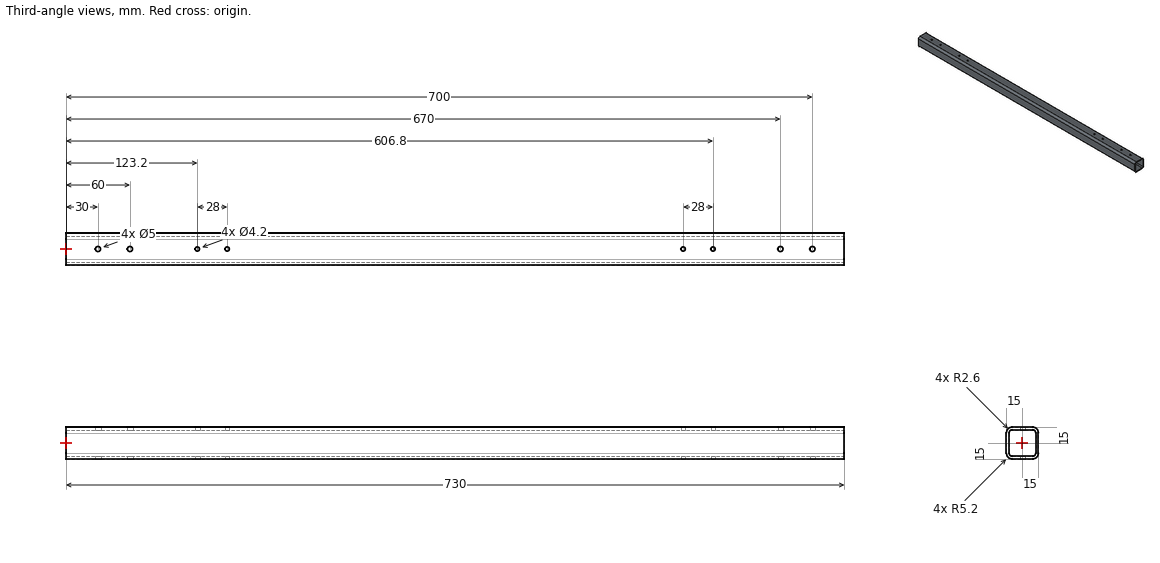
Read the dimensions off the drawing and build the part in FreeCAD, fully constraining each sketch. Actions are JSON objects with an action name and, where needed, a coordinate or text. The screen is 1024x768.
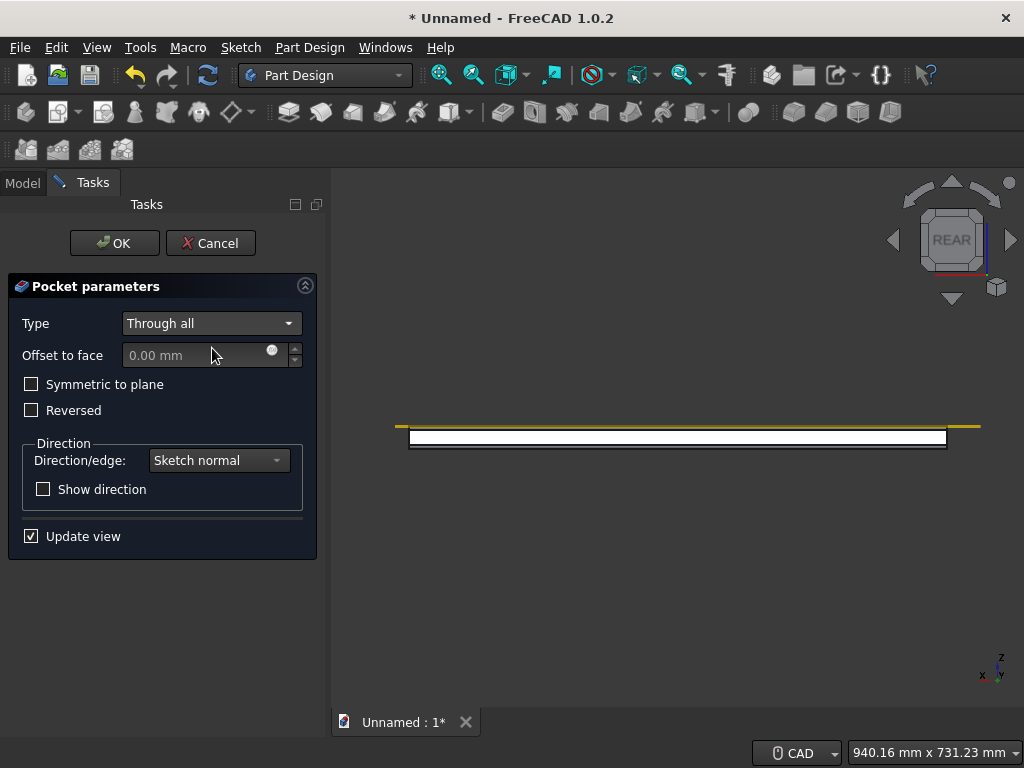
{"action": "left_click", "coordinate": [115, 243]}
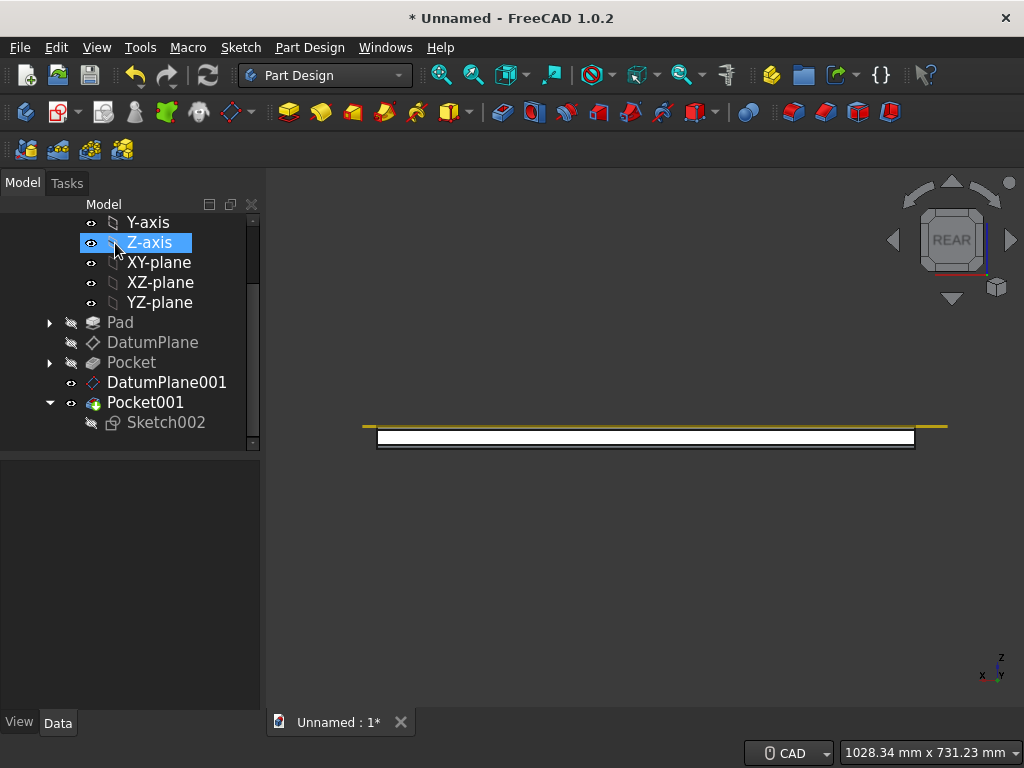
{"action": "left_click", "coordinate": [116, 383]}
{"action": "key", "text": "space"}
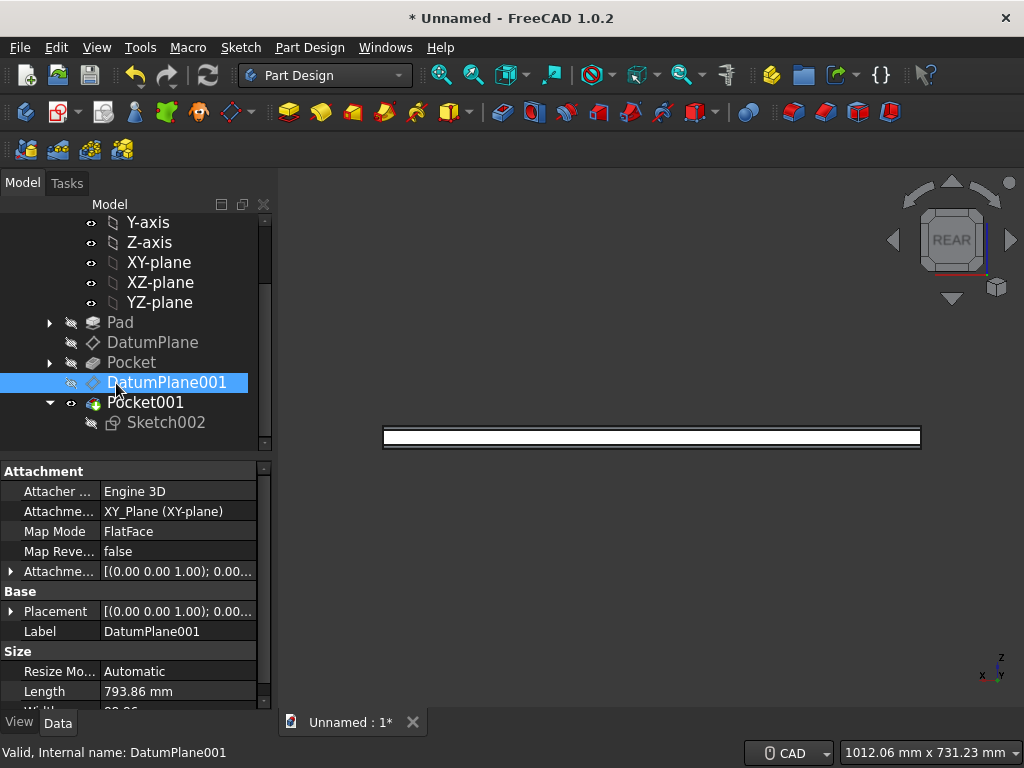
{"action": "key", "text": "0"}